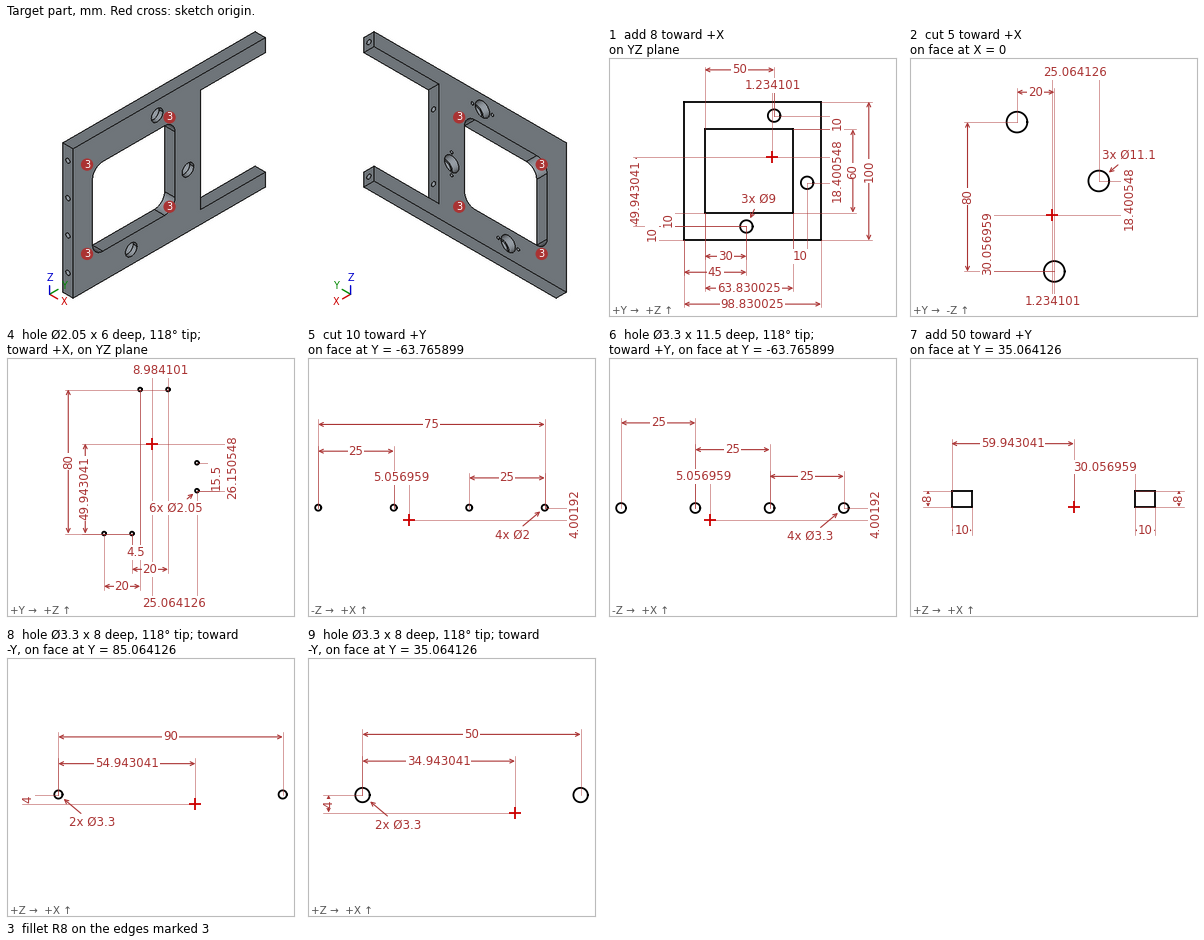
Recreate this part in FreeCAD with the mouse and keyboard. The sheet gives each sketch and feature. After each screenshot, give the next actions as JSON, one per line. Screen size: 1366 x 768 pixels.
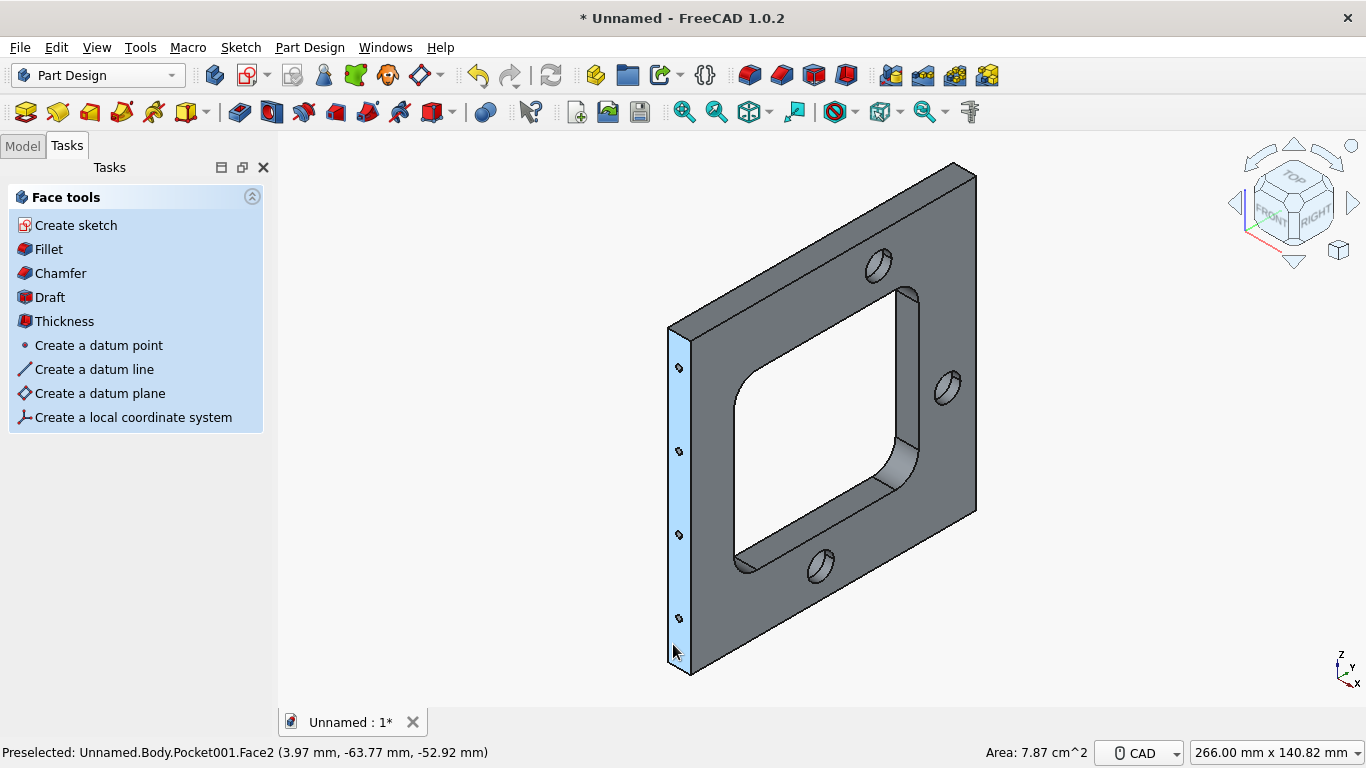
{"action": "left_click", "coordinate": [248, 76]}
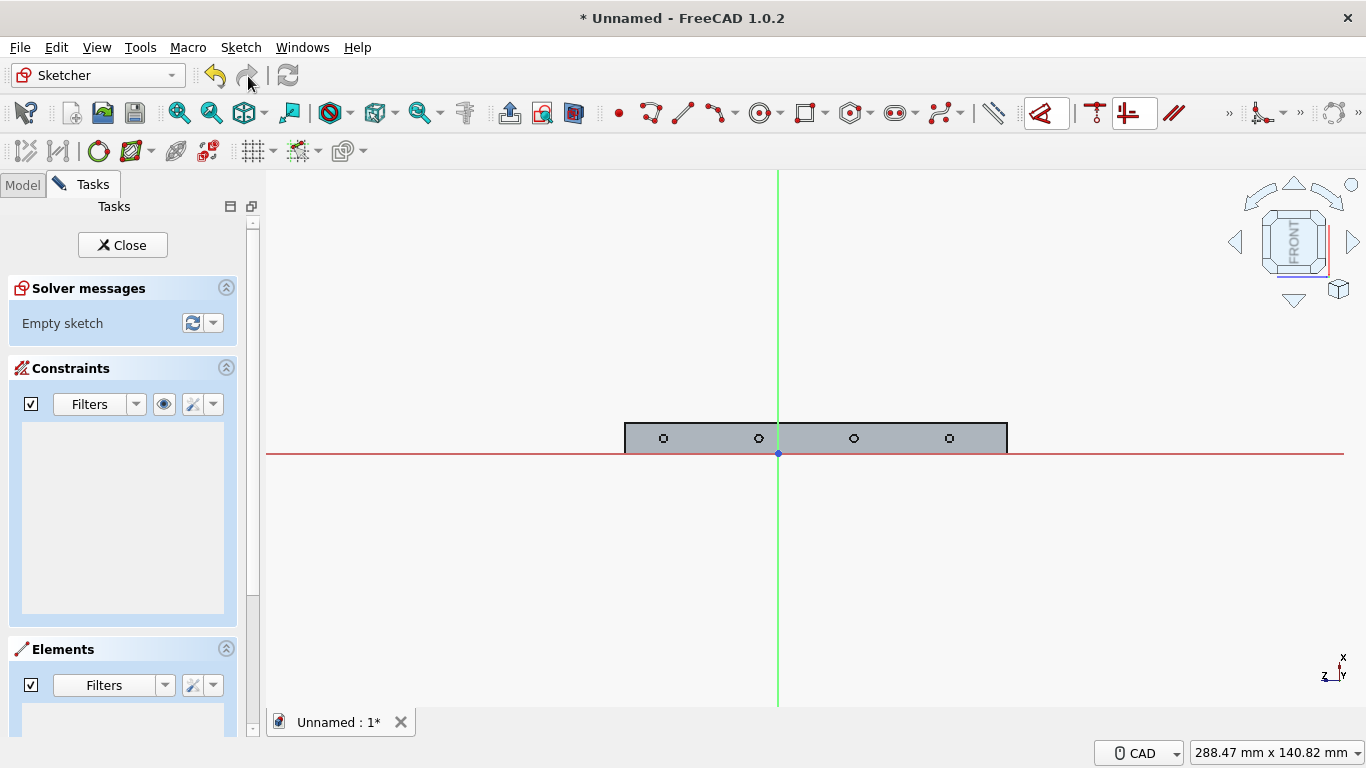
{"action": "scroll", "coordinate": [855, 447], "scroll_direction": "up", "scroll_amount": 4}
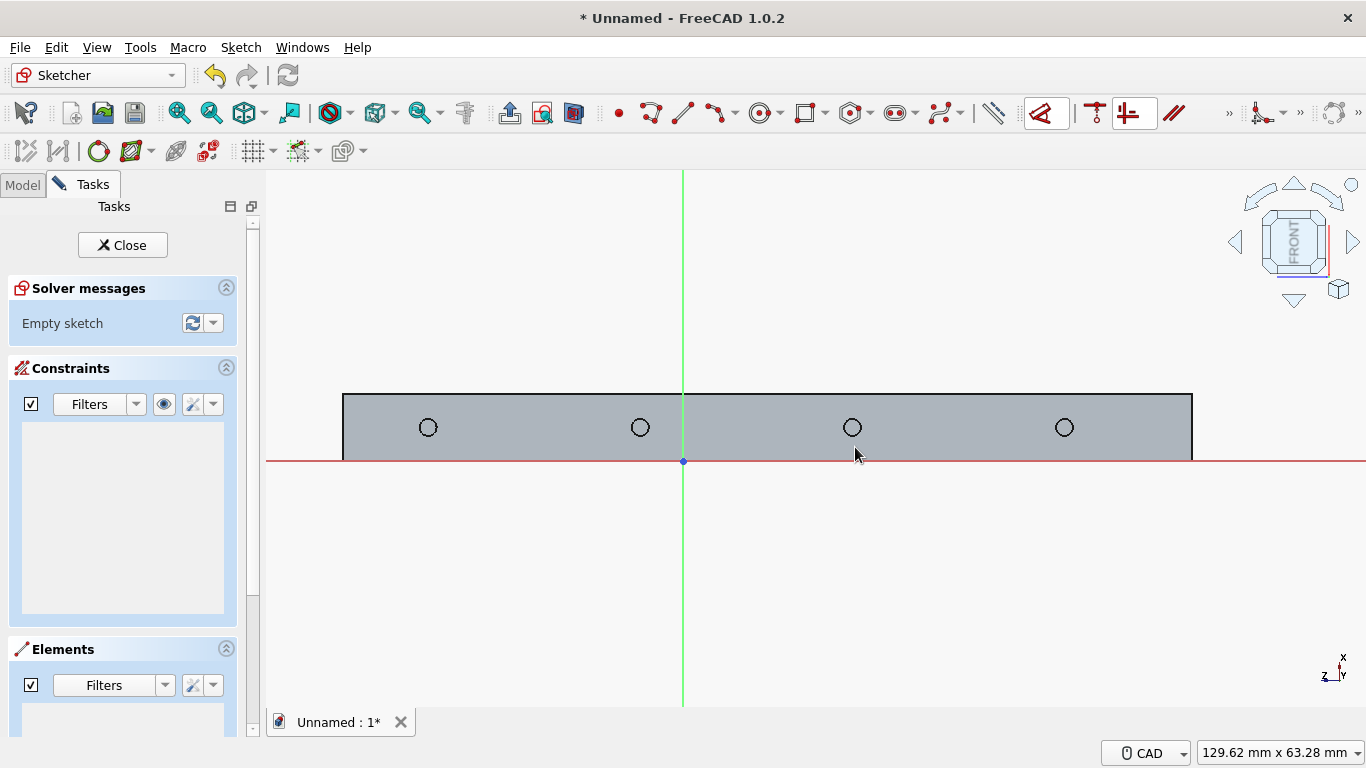
{"action": "left_click", "coordinate": [760, 114]}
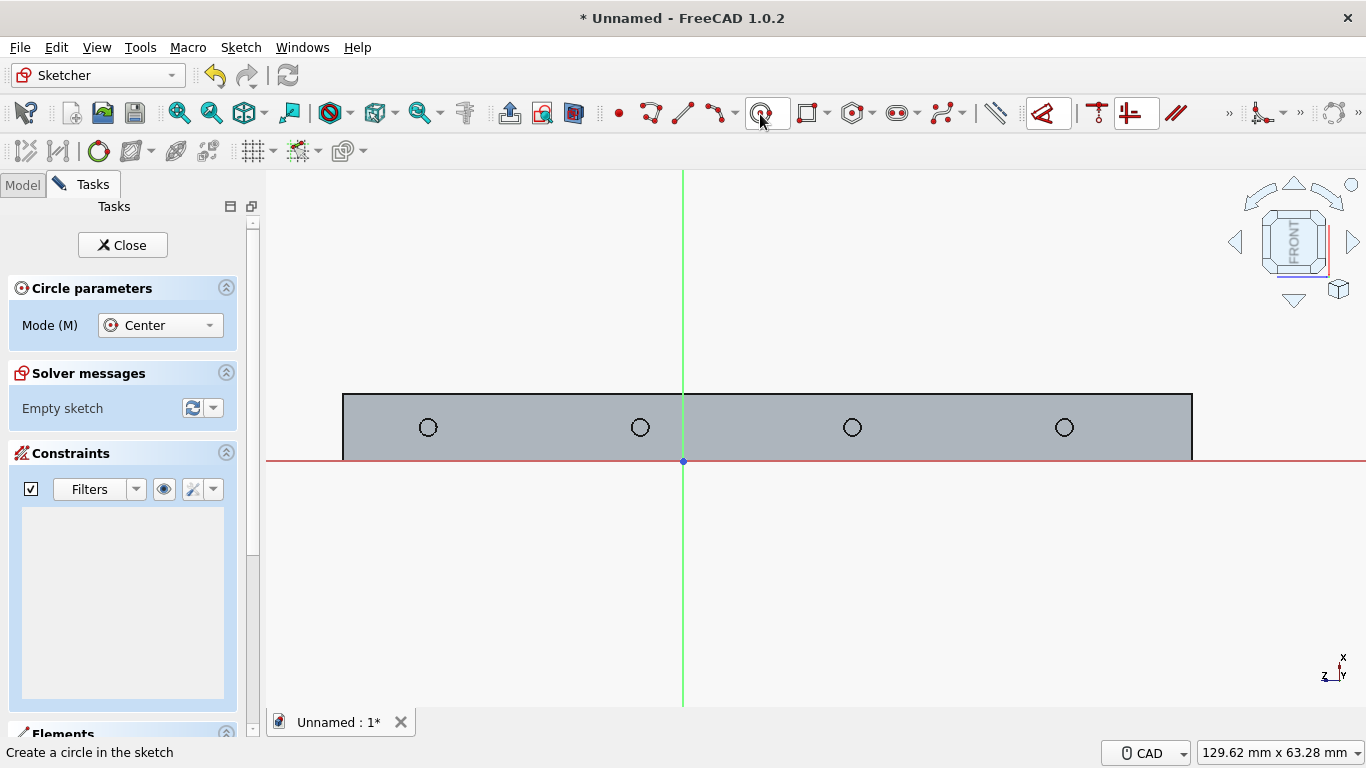
{"action": "scroll", "coordinate": [1065, 427], "scroll_direction": "up", "scroll_amount": 3}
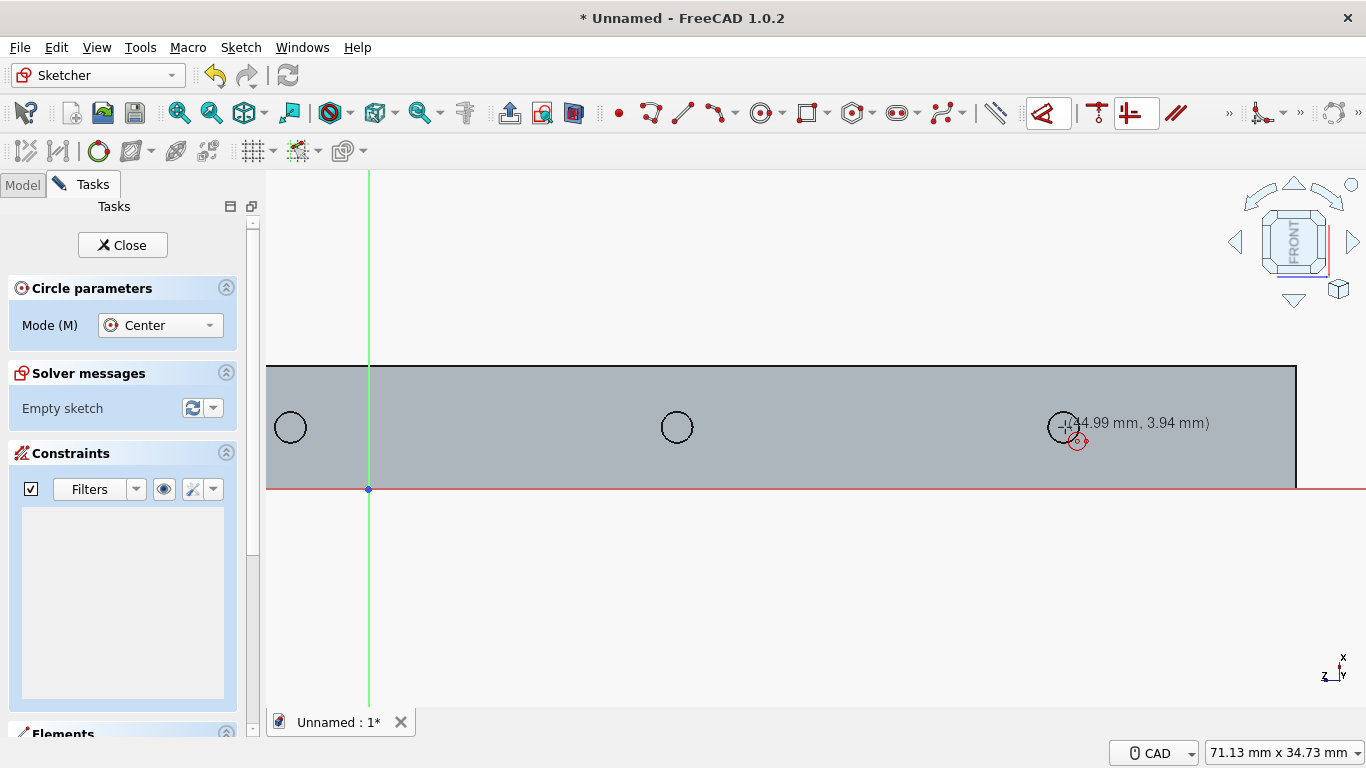
{"action": "left_click", "coordinate": [1064, 427]}
{"action": "mouse_move", "coordinate": [1082, 409]}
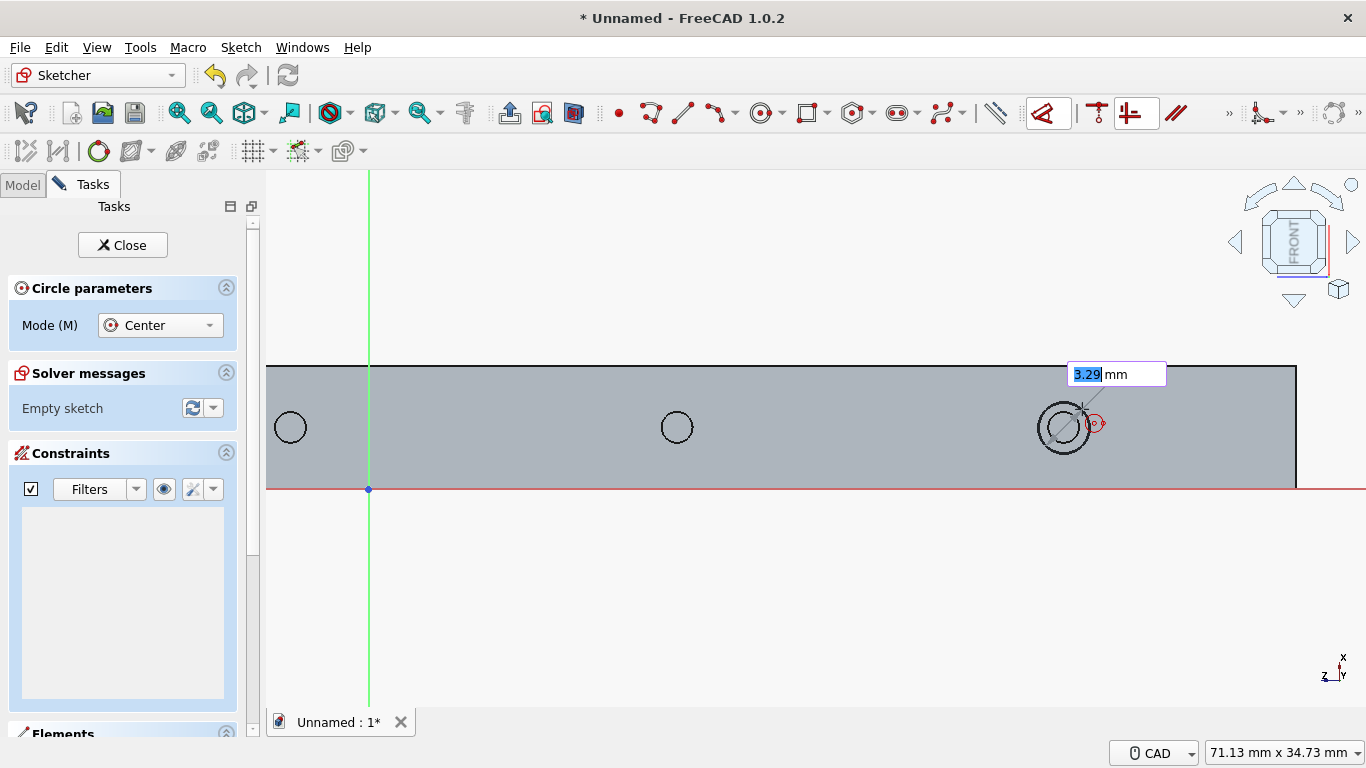
{"action": "type", "text": "3.3"}
{"action": "key", "text": "Return"}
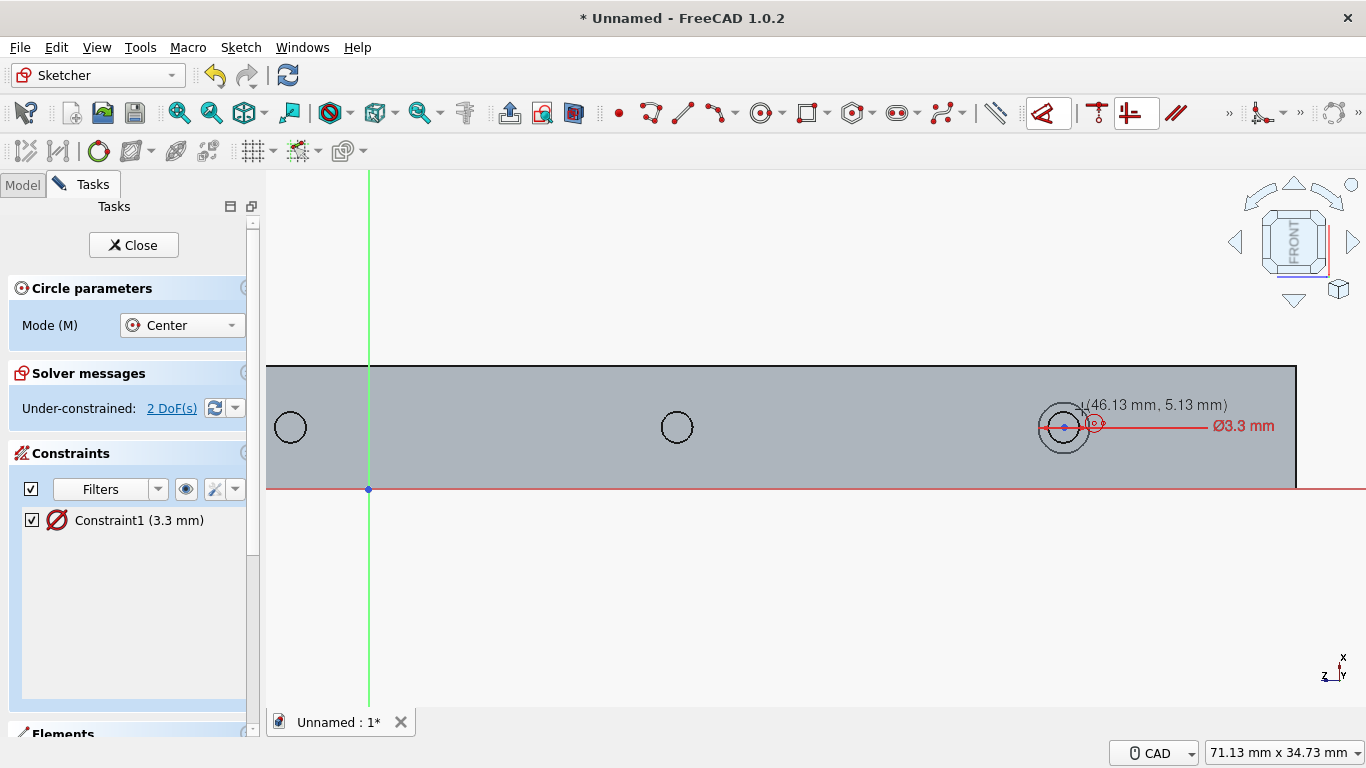
{"action": "left_click", "coordinate": [677, 427]}
{"action": "mouse_move", "coordinate": [695, 409]}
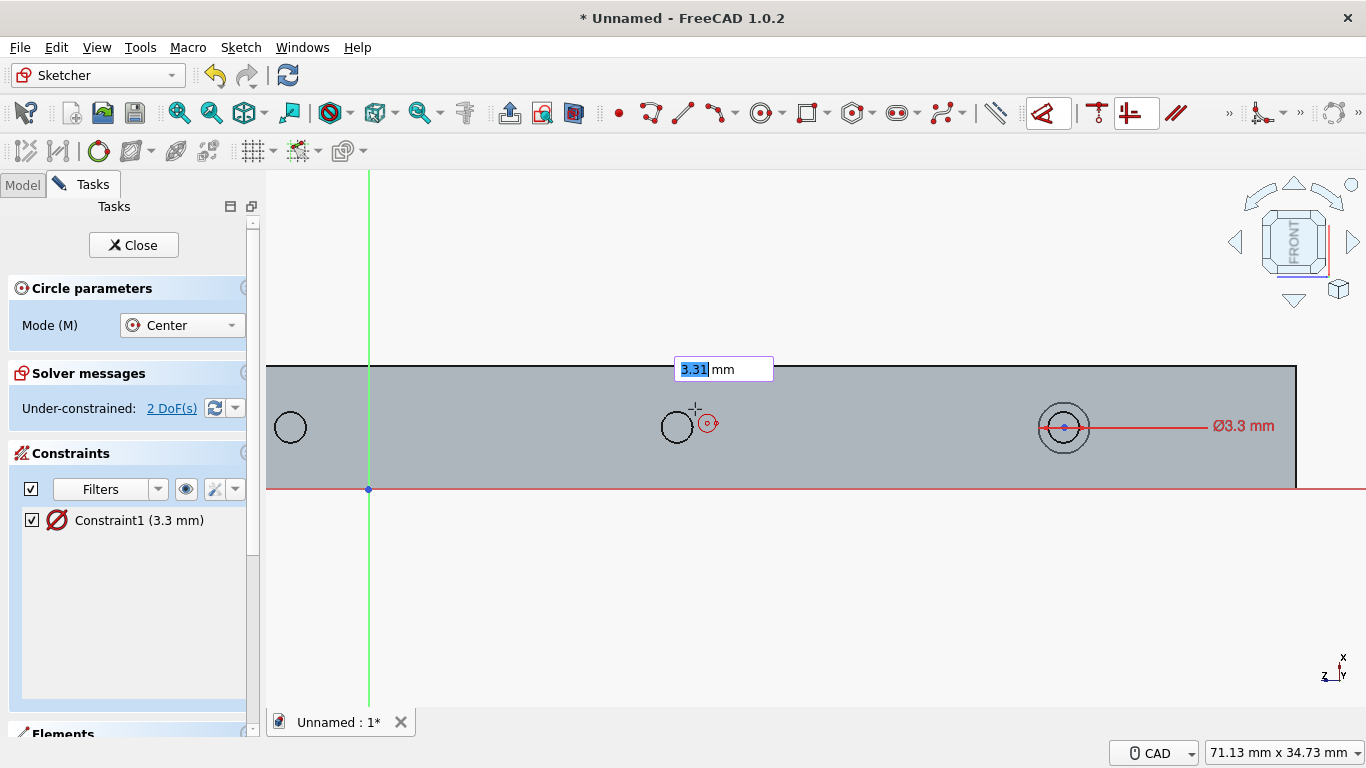
{"action": "type", "text": "3.3"}
{"action": "key", "text": "Return"}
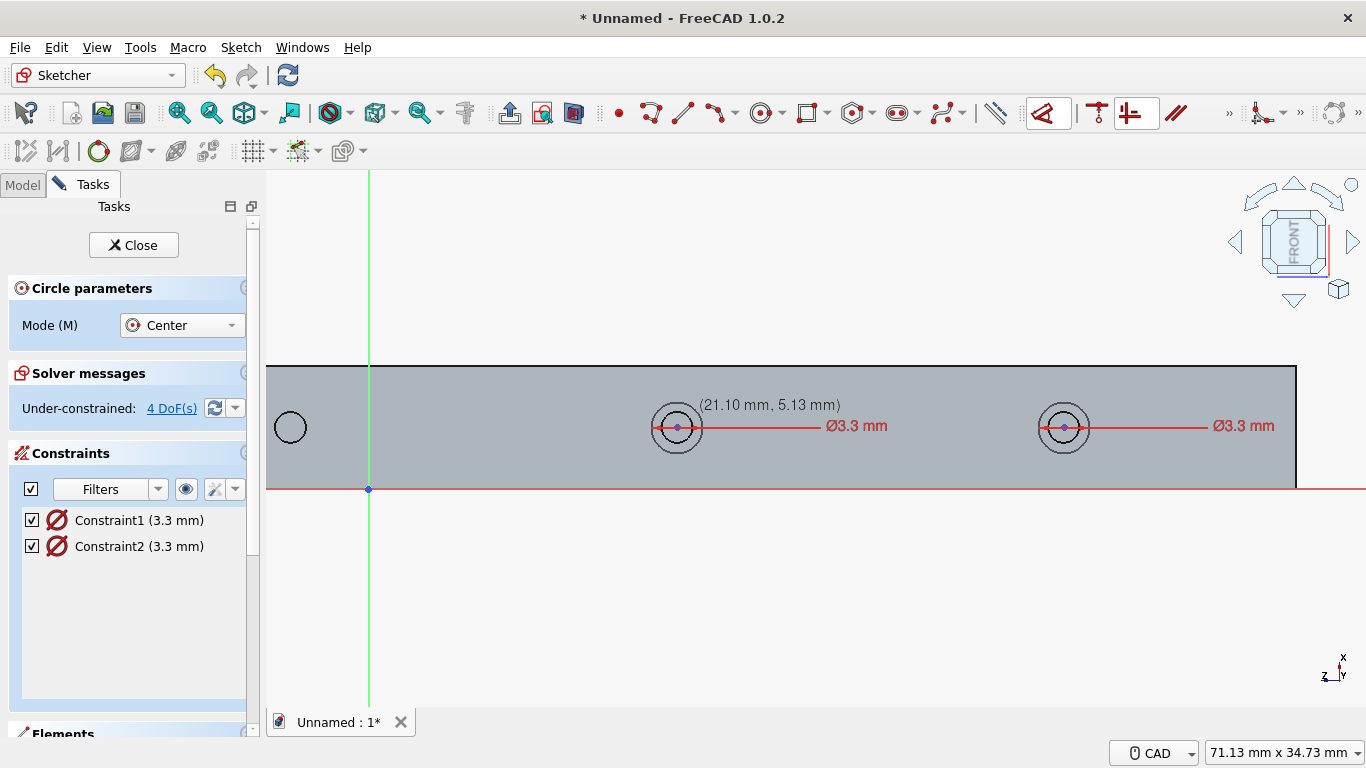
{"action": "scroll", "coordinate": [1068, 430], "scroll_direction": "down", "scroll_amount": 3}